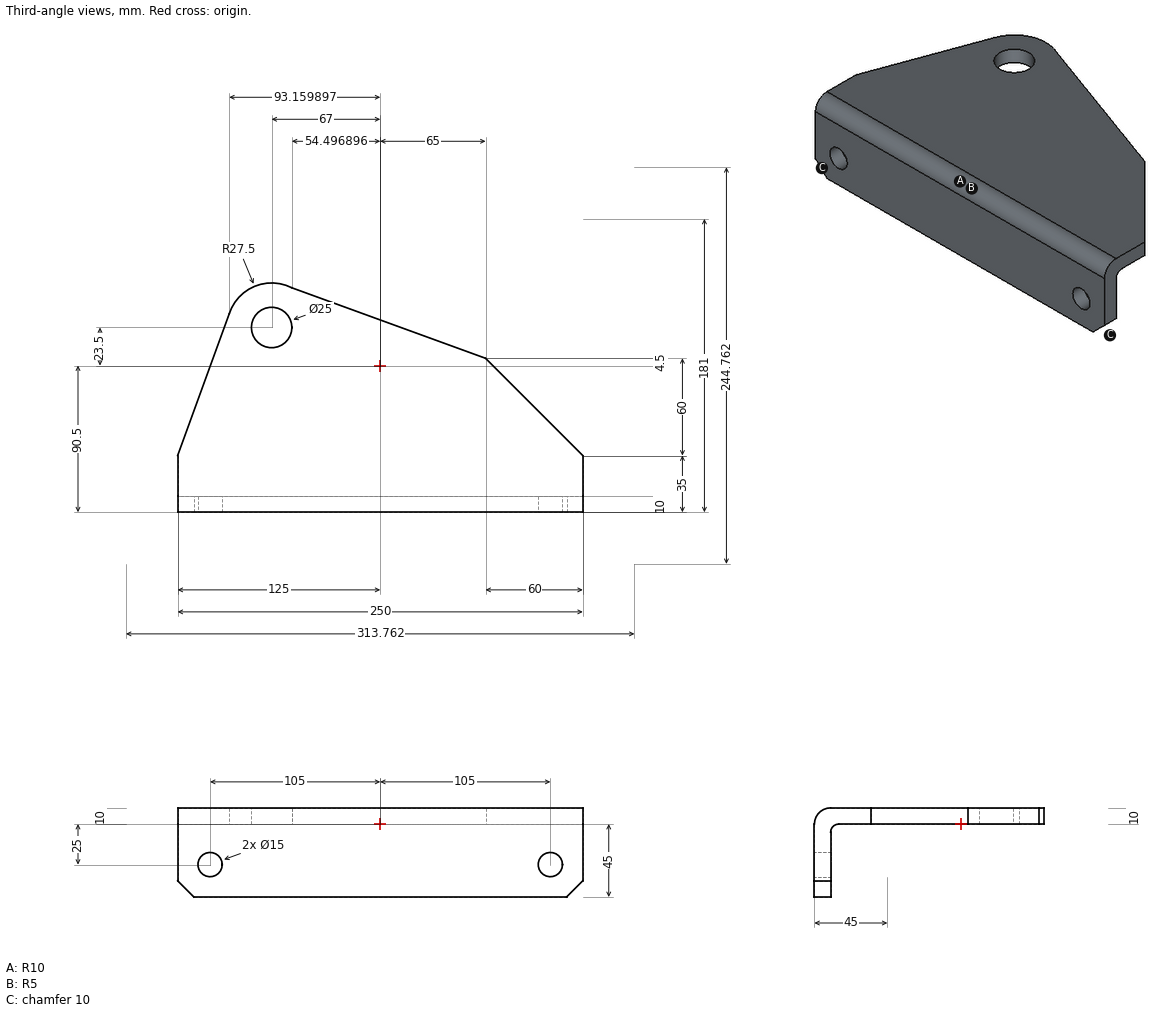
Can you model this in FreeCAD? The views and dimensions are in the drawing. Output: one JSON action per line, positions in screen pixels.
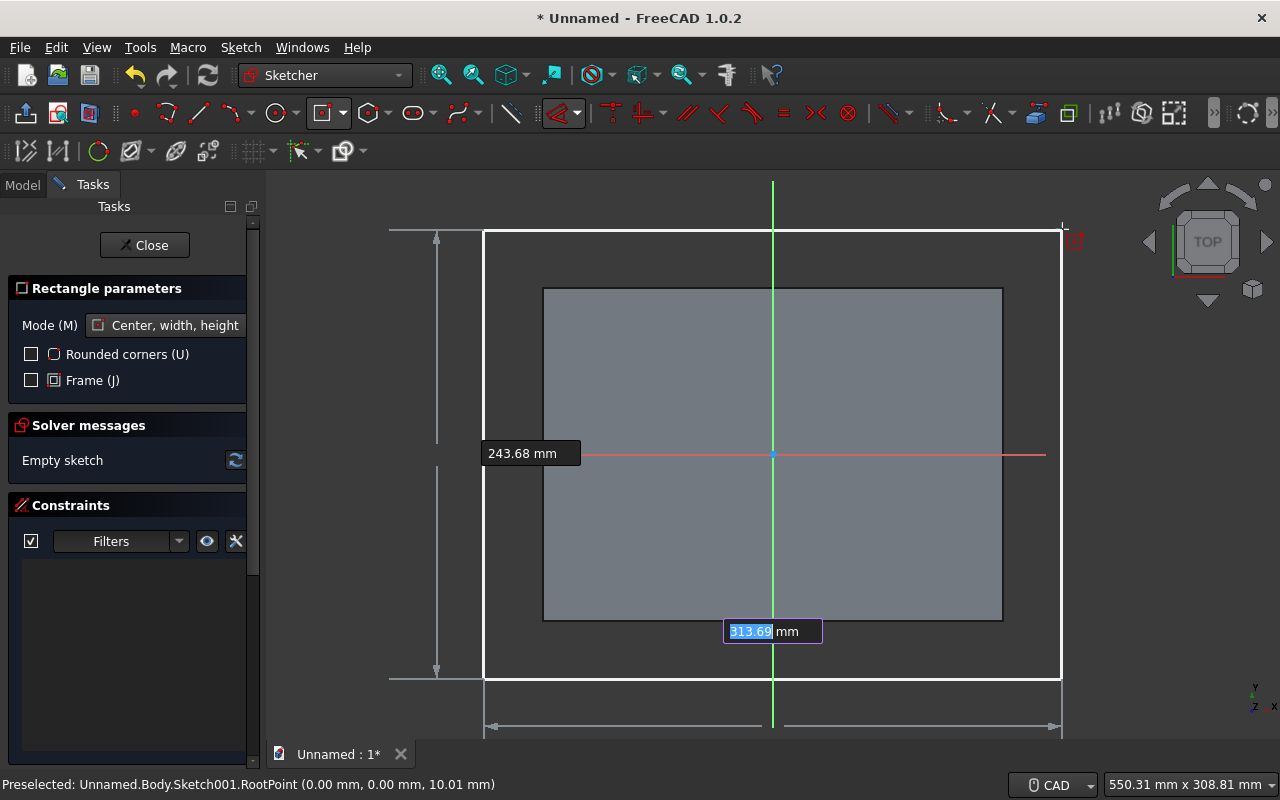
{"action": "type", "text": "313.762"}
{"action": "key", "text": "Tab"}
{"action": "type", "text": "244.762"}
{"action": "key", "text": "Return"}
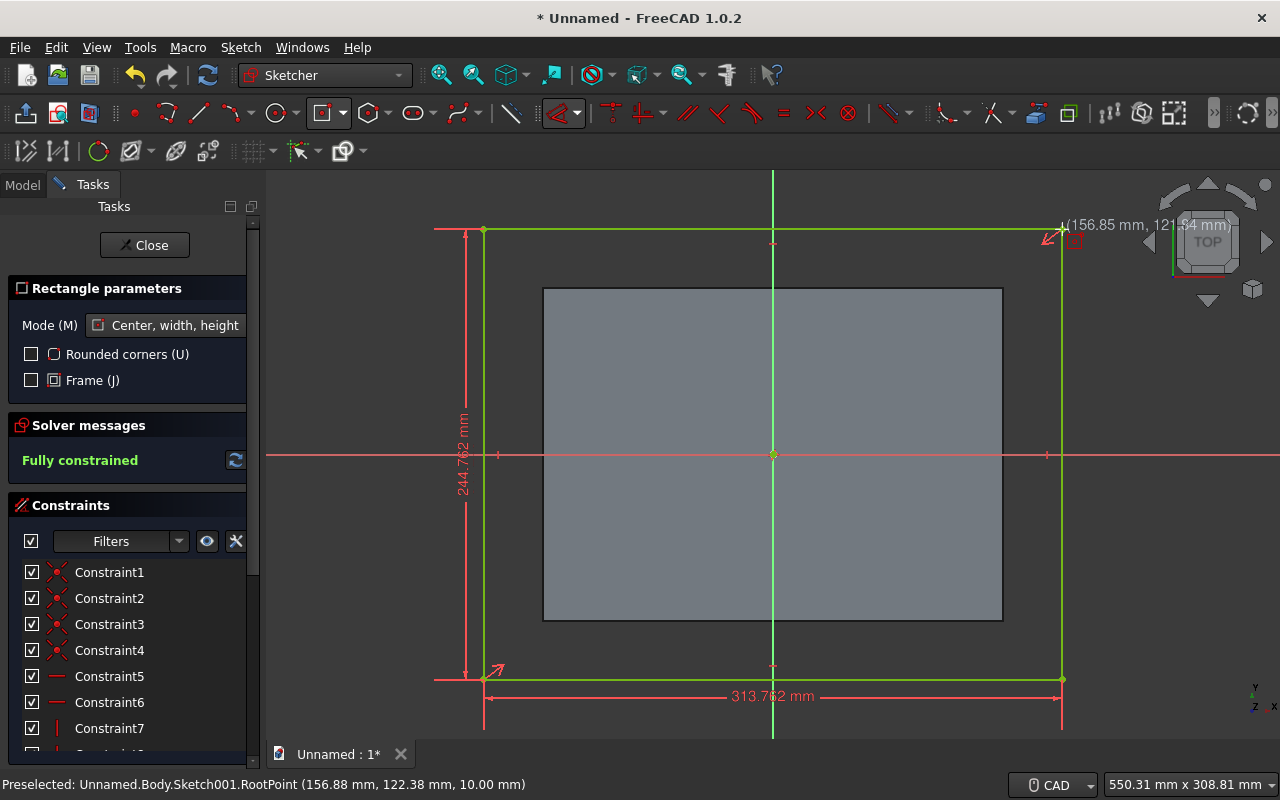
{"action": "key", "text": "g m"}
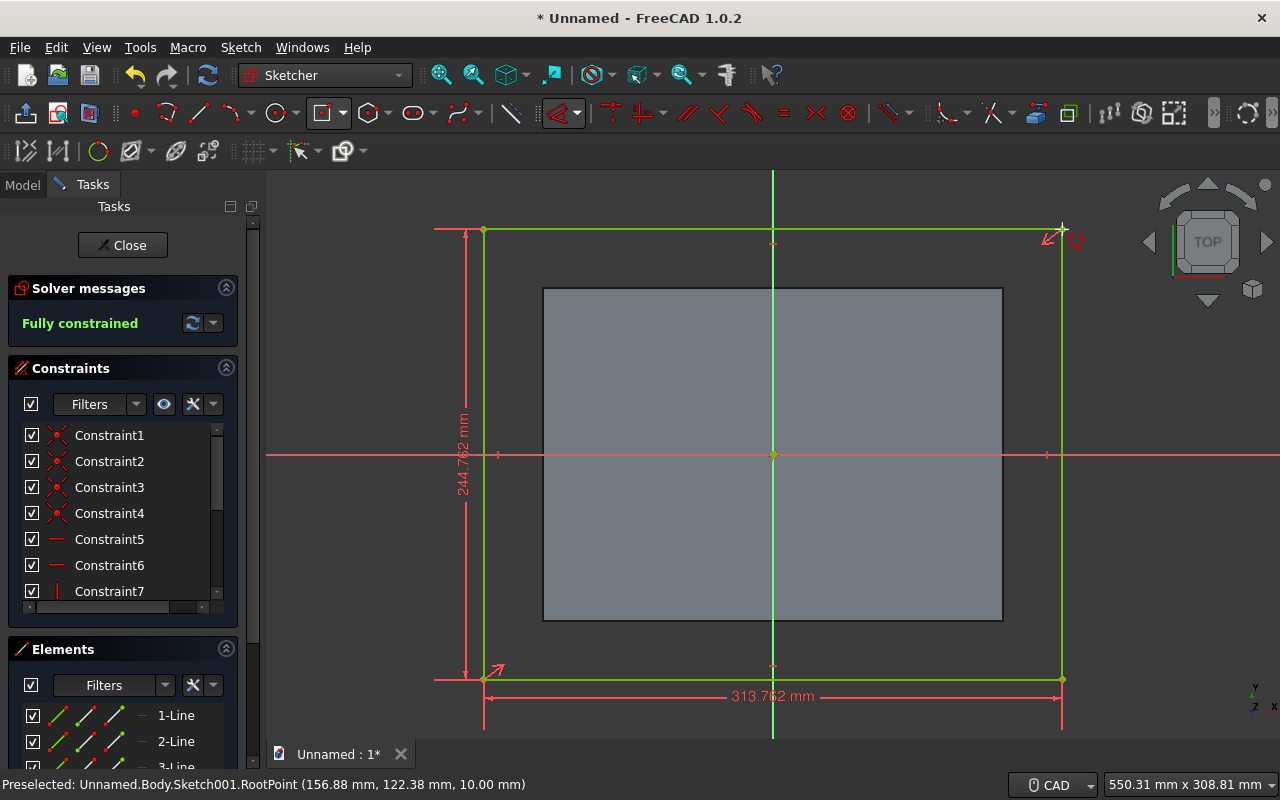
{"action": "left_click", "coordinate": [673, 366]}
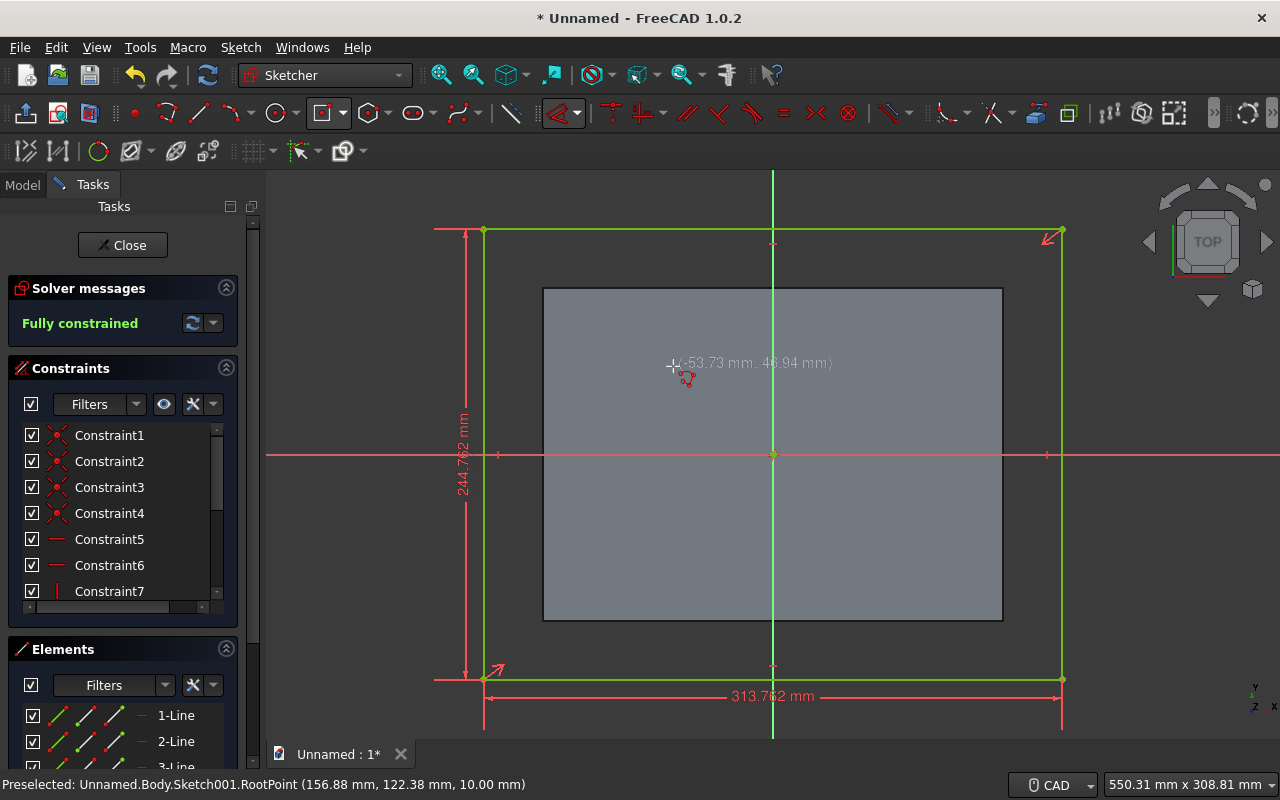
{"action": "scroll", "coordinate": [893, 446], "scroll_direction": "up", "scroll_amount": 4}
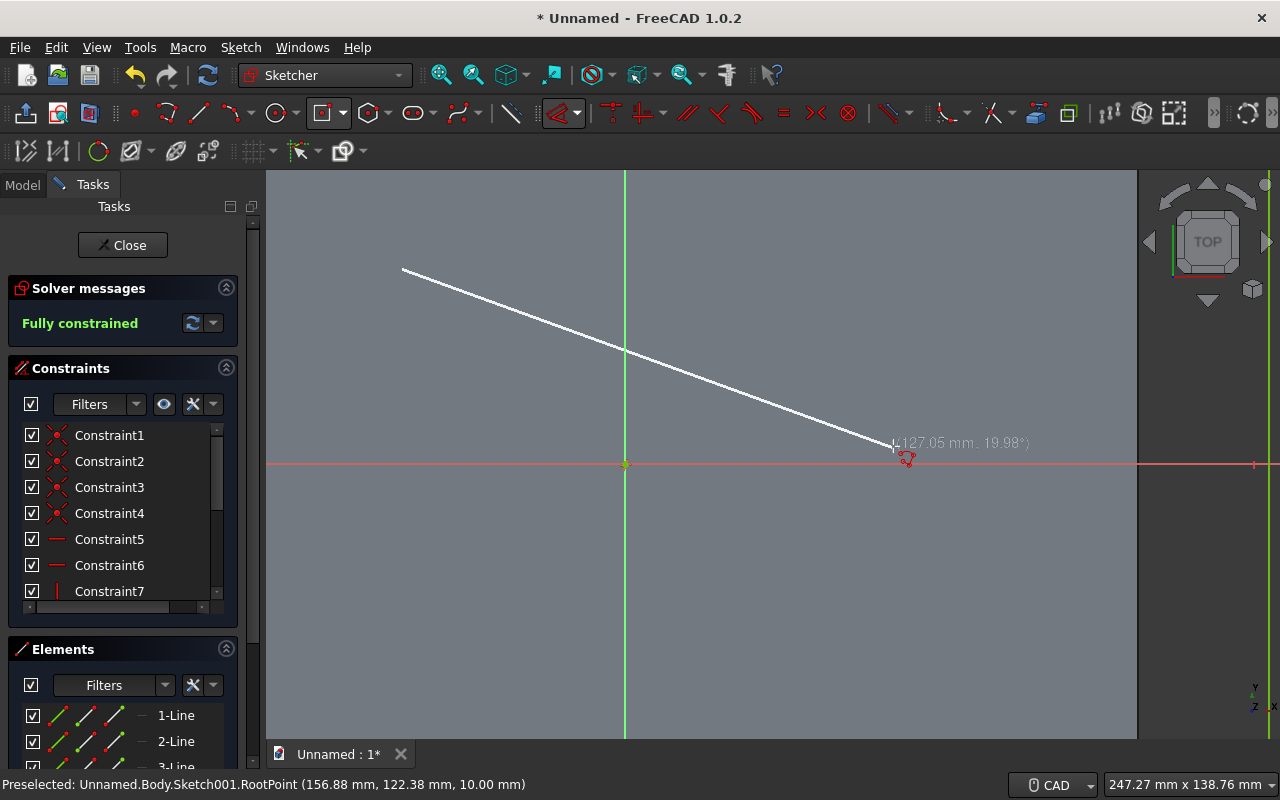
{"action": "left_click", "coordinate": [892, 446]}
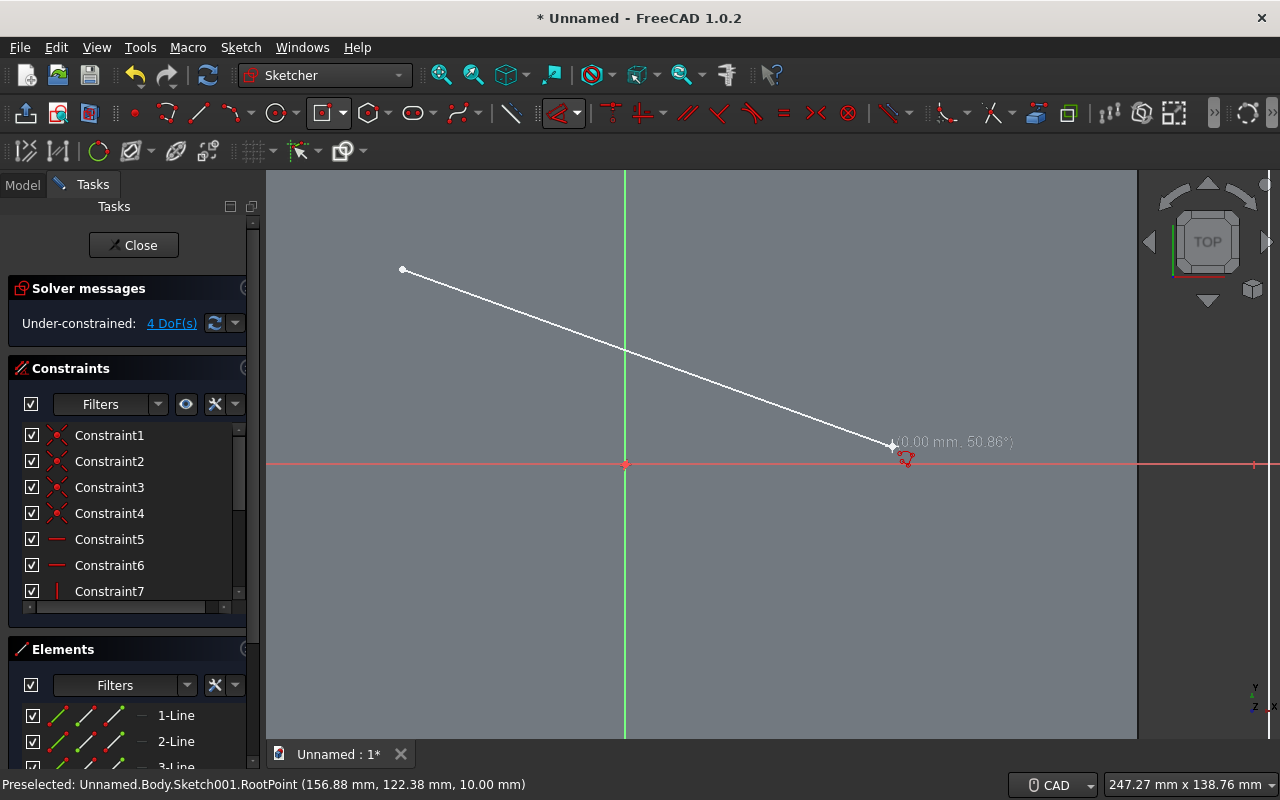
{"action": "scroll", "coordinate": [751, 449], "scroll_direction": "down", "scroll_amount": 5}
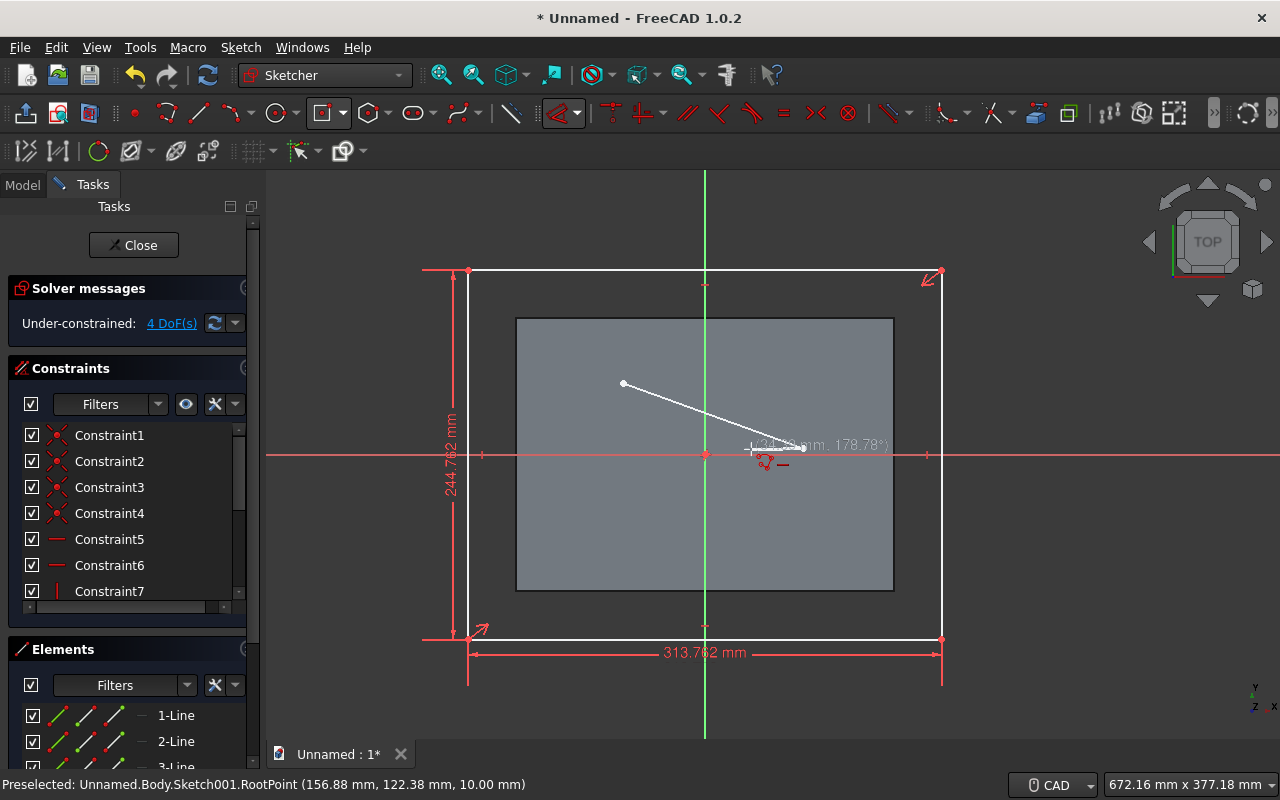
{"action": "left_click", "coordinate": [894, 539]}
{"action": "left_click", "coordinate": [894, 591]}
{"action": "left_click", "coordinate": [516, 591]}
{"action": "left_click", "coordinate": [516, 539]}
{"action": "left_click", "coordinate": [564, 407]}
{"action": "right_click", "coordinate": [564, 407]}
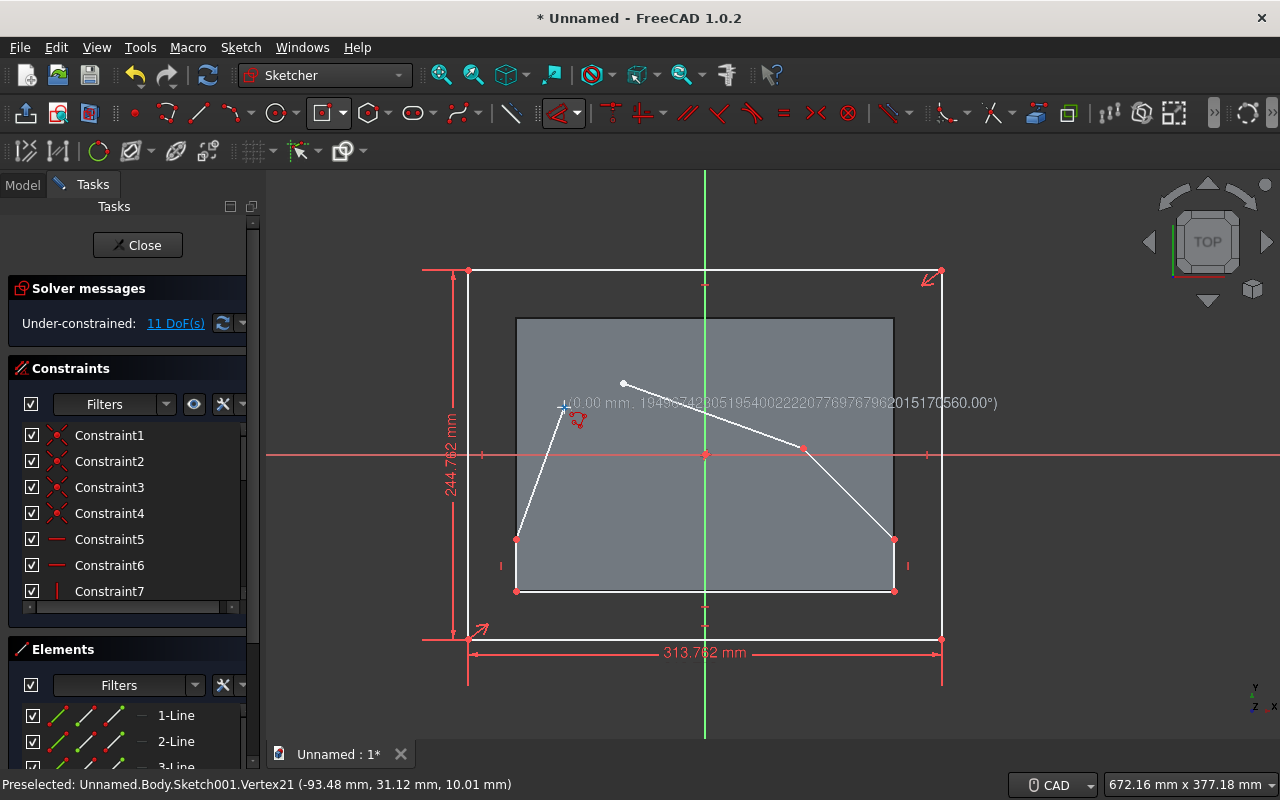
{"action": "left_click", "coordinate": [232, 114]}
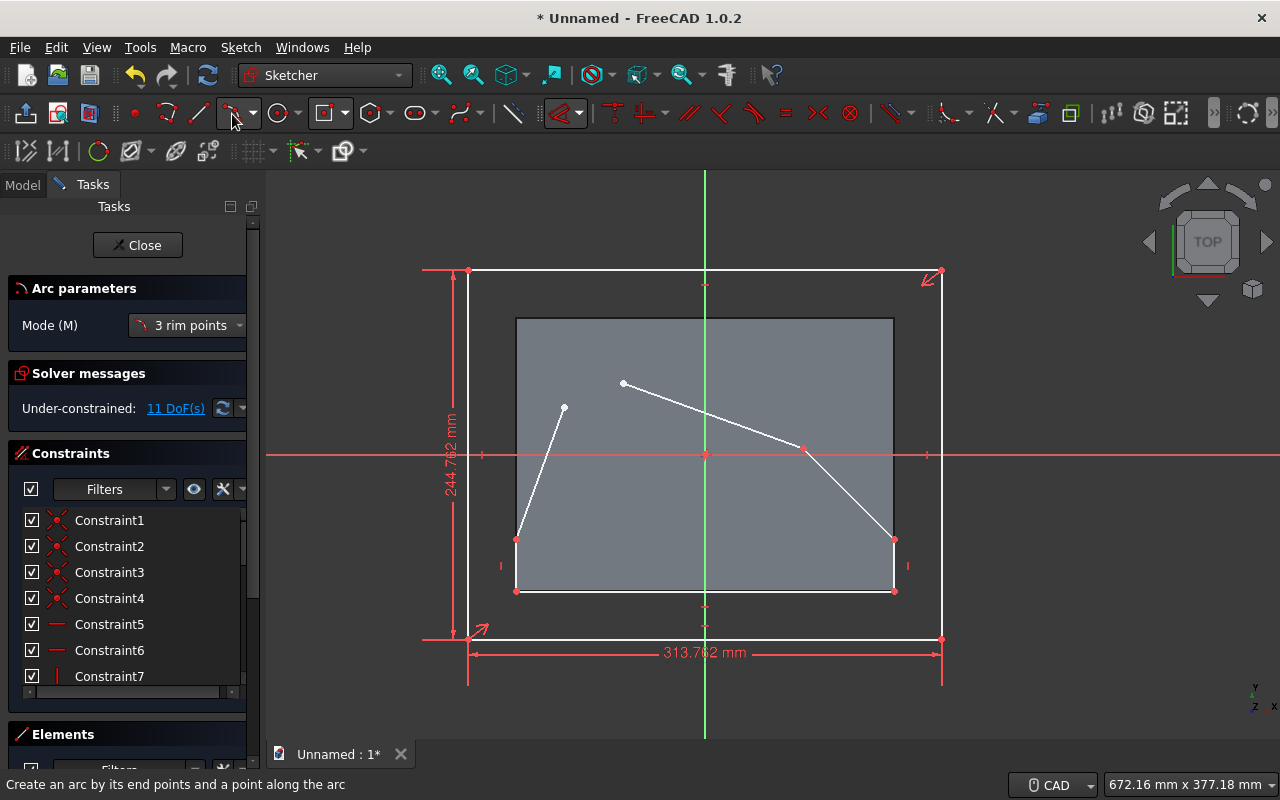
{"action": "left_click", "coordinate": [564, 408]}
{"action": "left_click", "coordinate": [623, 383]}
{"action": "left_click", "coordinate": [588, 381]}
{"action": "key", "text": "Escape"}